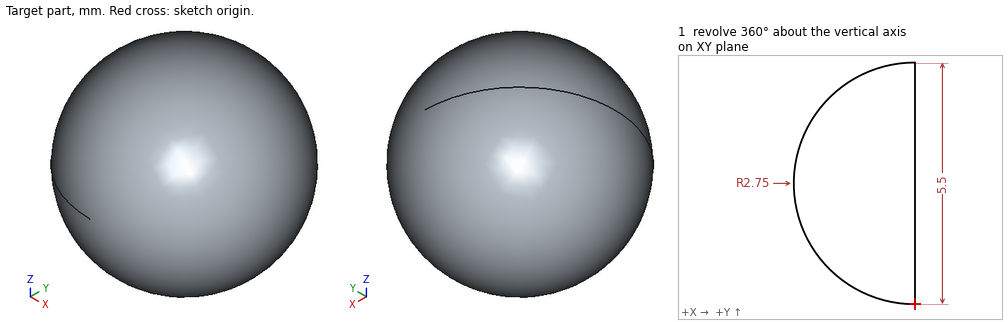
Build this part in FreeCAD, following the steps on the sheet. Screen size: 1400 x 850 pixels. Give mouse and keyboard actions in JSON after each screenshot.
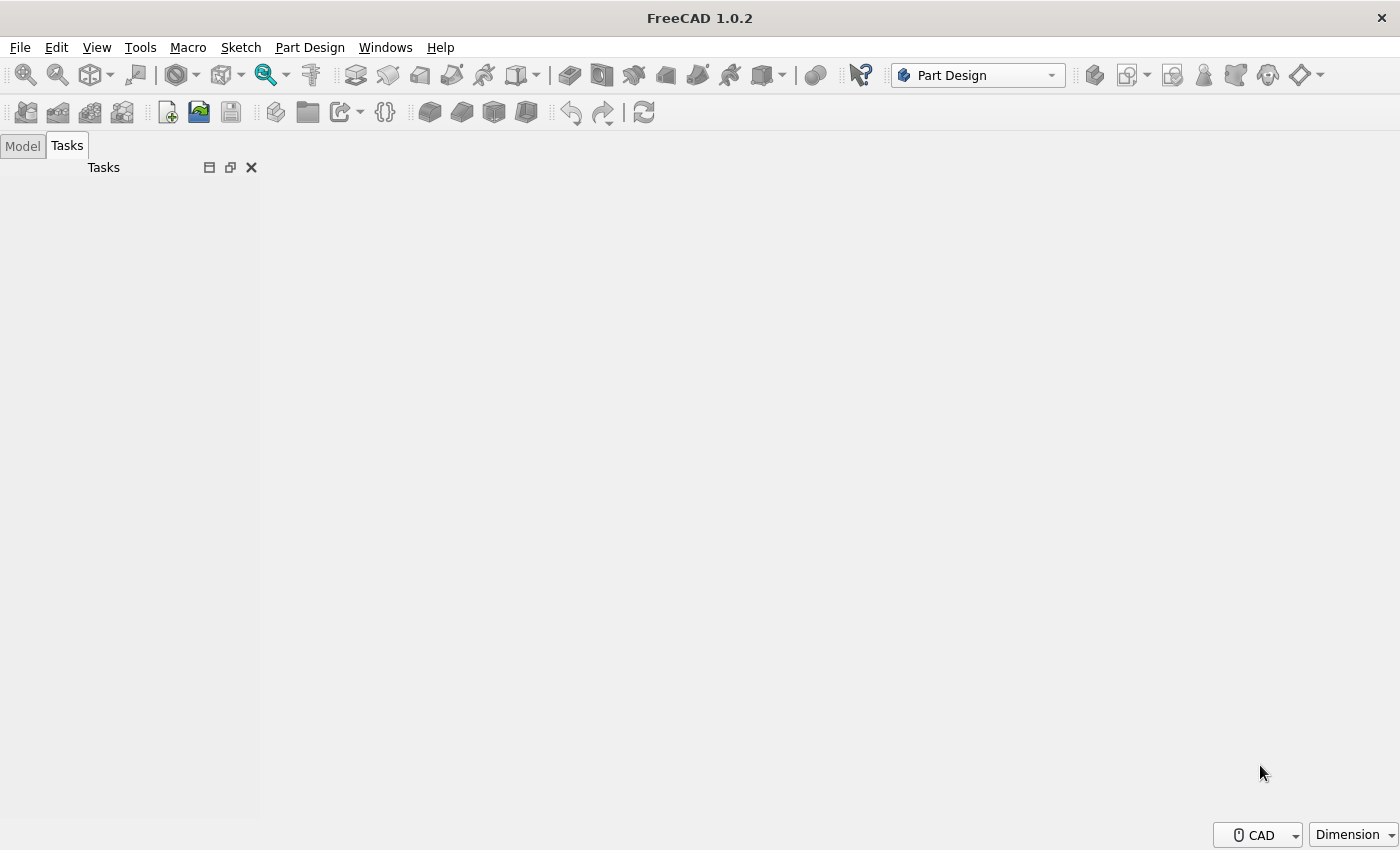
{"action": "left_click", "coordinate": [168, 112]}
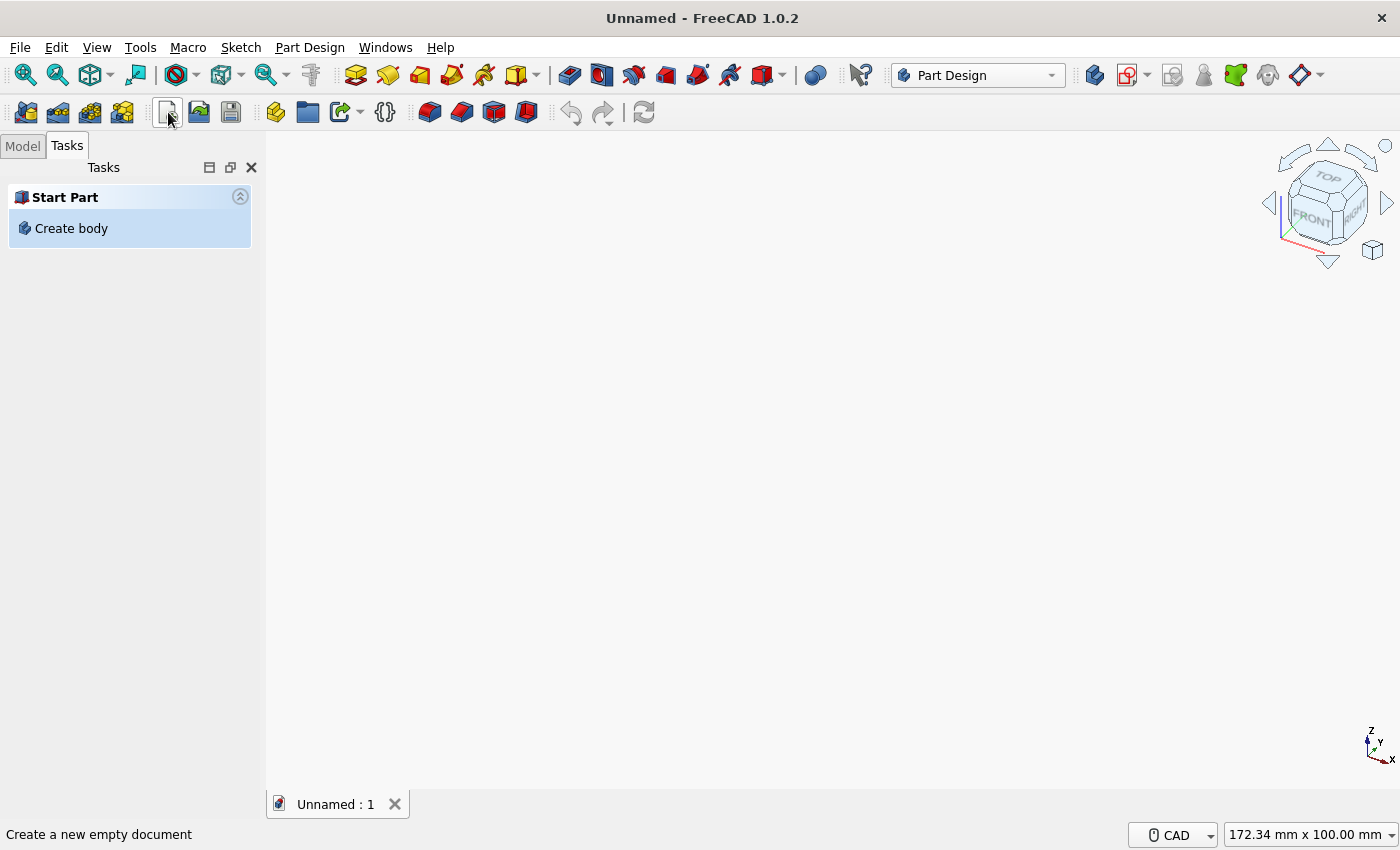
{"action": "left_click", "coordinate": [1128, 76]}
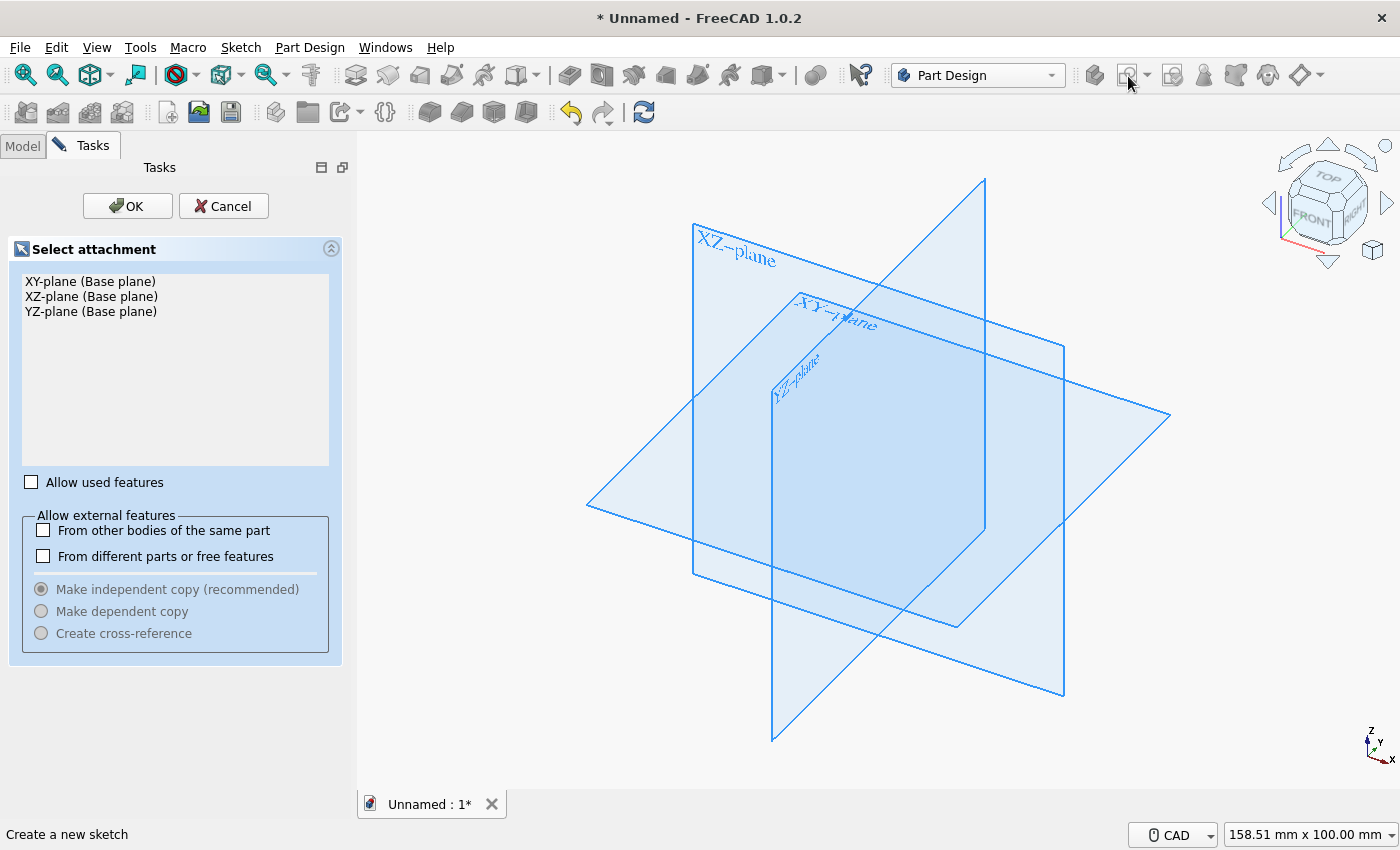
{"action": "left_click", "coordinate": [82, 282]}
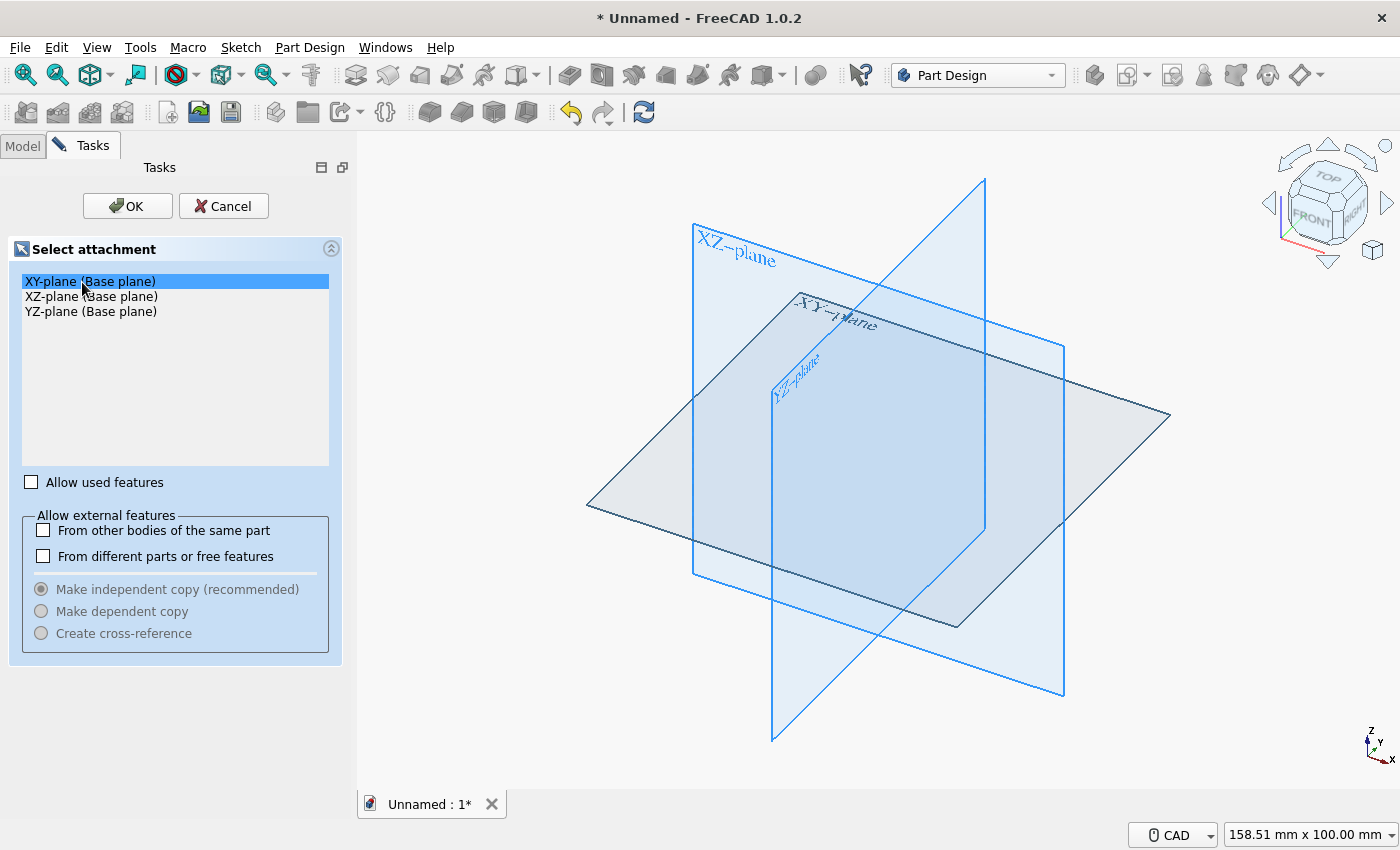
{"action": "left_click", "coordinate": [128, 206]}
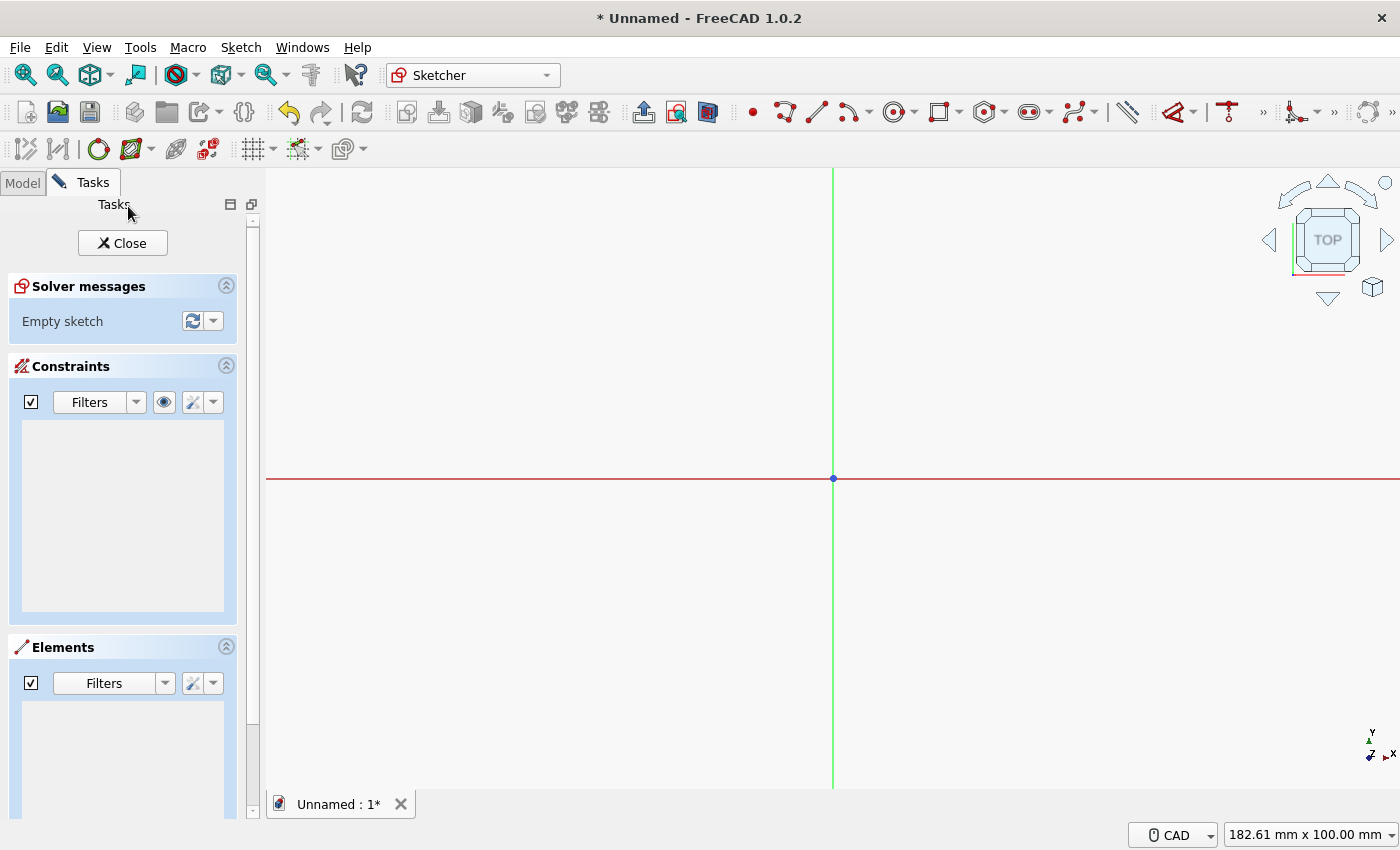
{"action": "scroll", "coordinate": [830, 460], "scroll_direction": "up", "scroll_amount": 12}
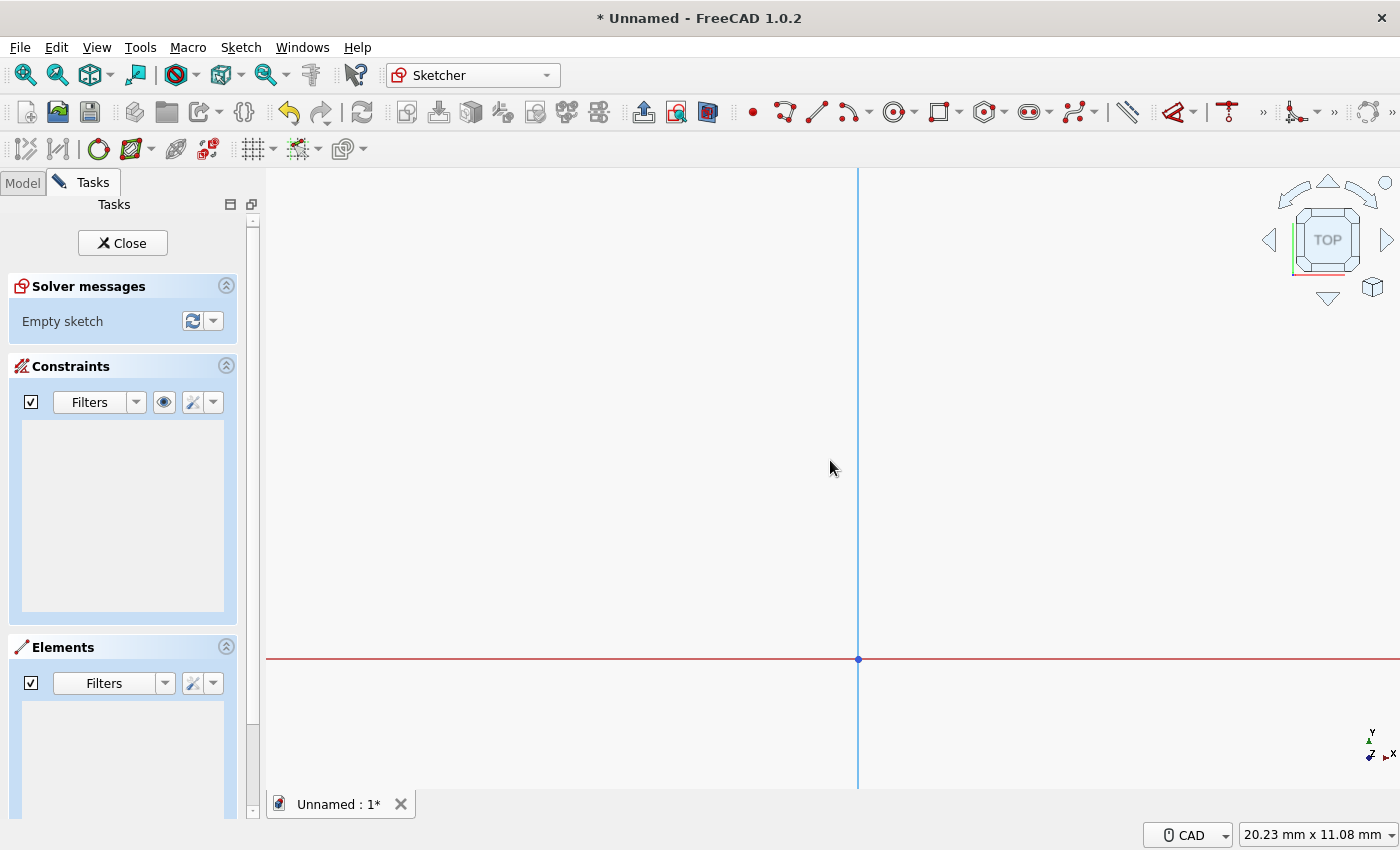
{"action": "left_click", "coordinate": [818, 112]}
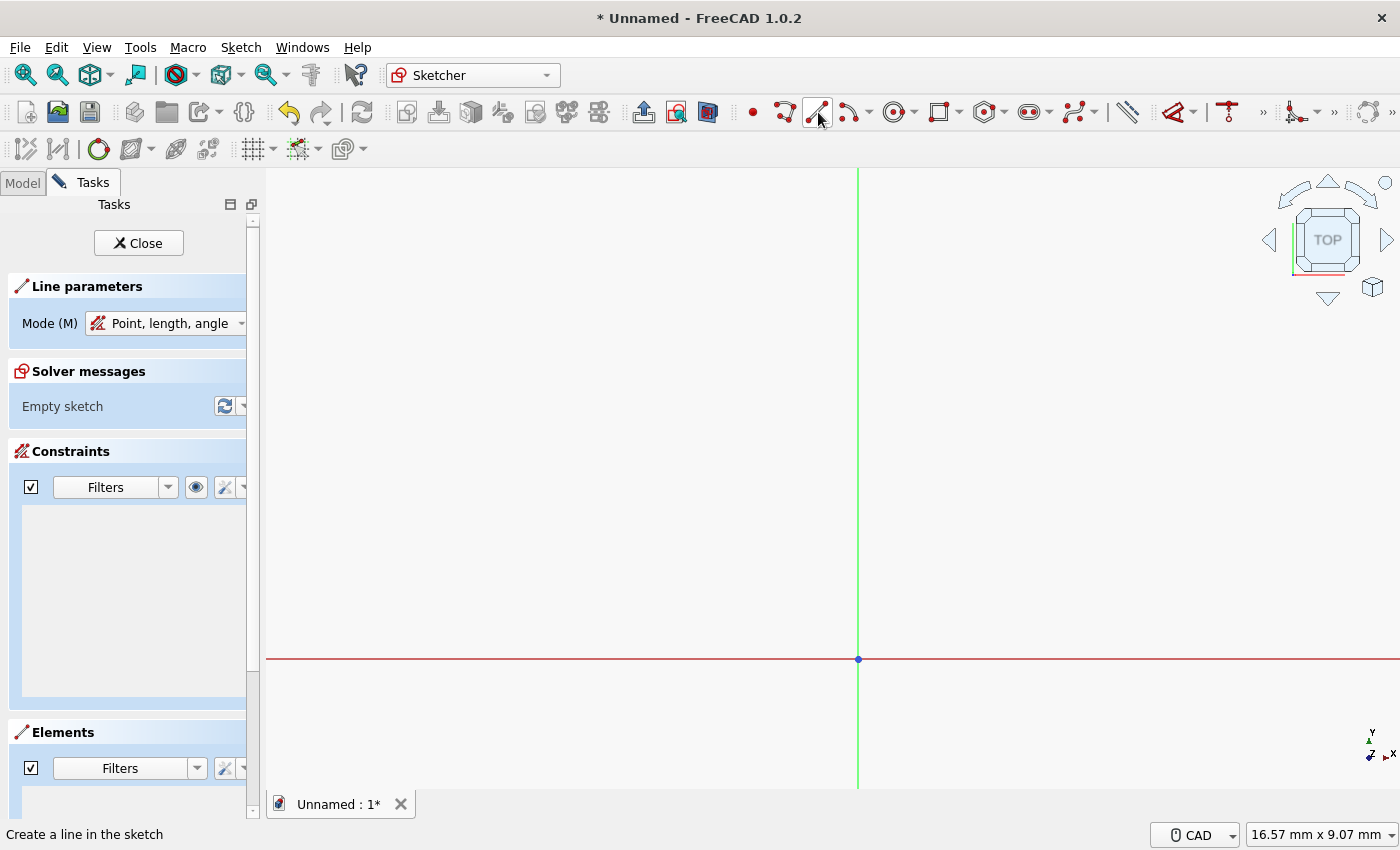
{"action": "left_click", "coordinate": [858, 659]}
{"action": "left_click", "coordinate": [849, 283]}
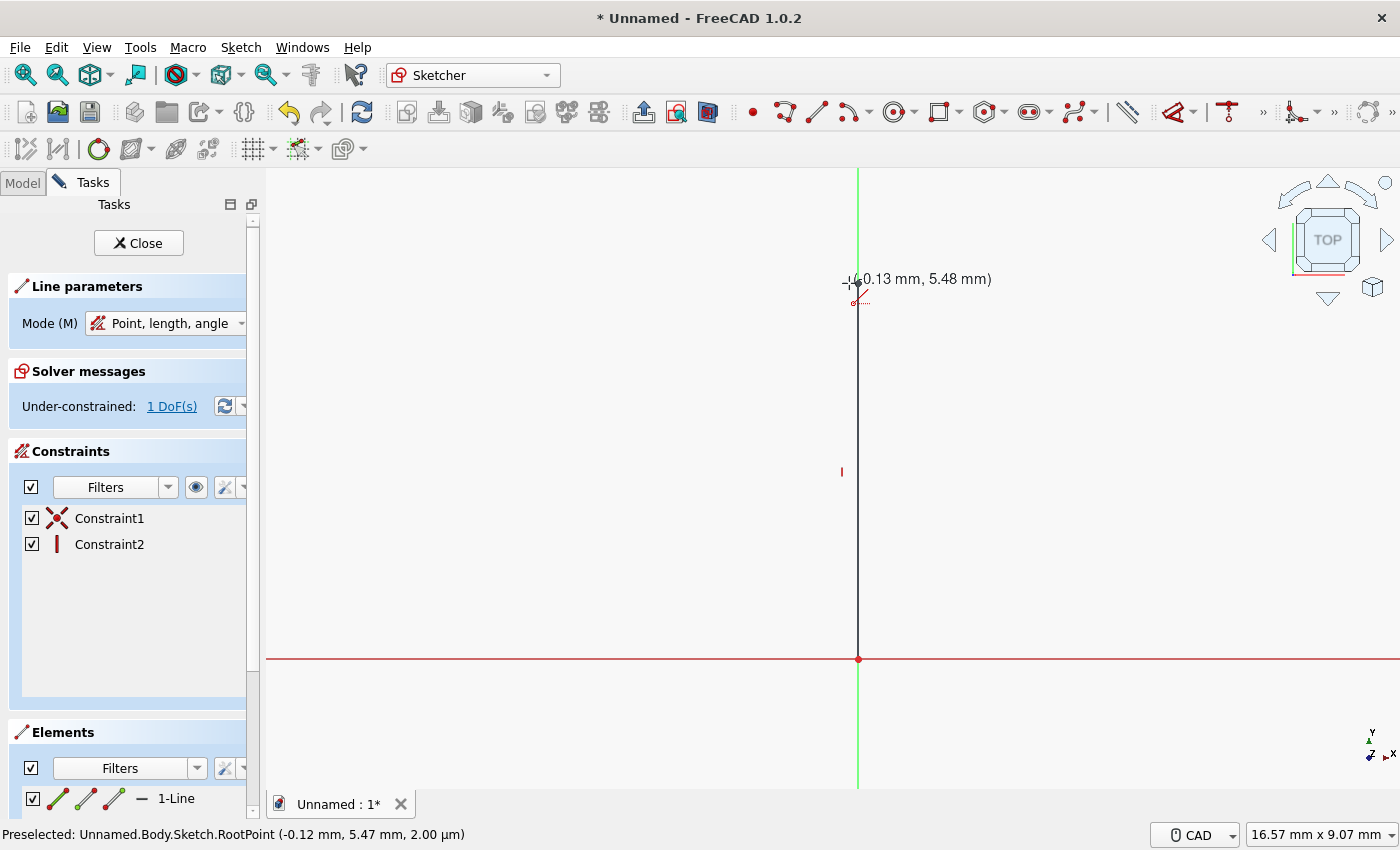
{"action": "key", "text": "g 3 a"}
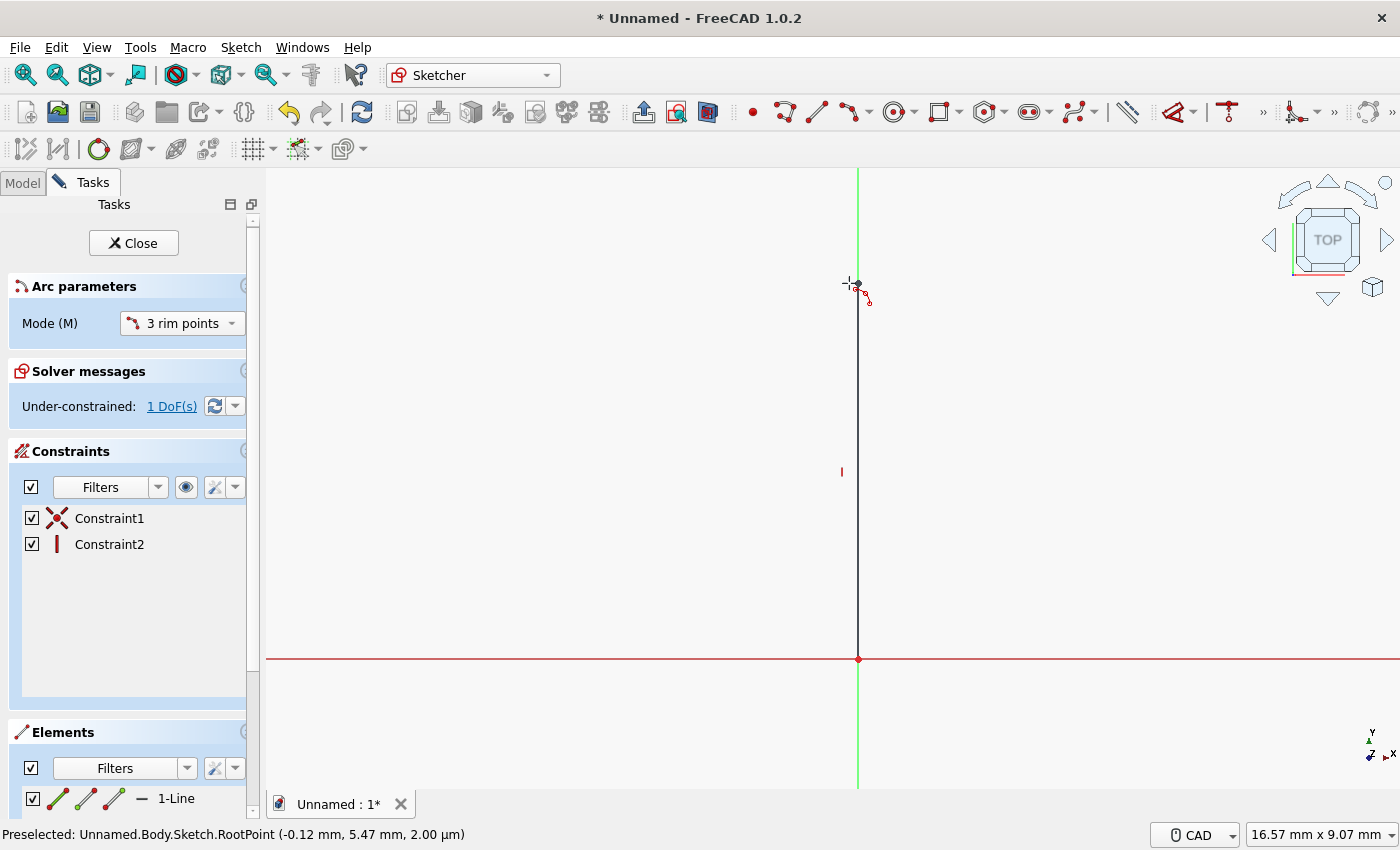
{"action": "left_click", "coordinate": [849, 283]}
{"action": "left_click", "coordinate": [858, 659]}
{"action": "left_click", "coordinate": [670, 471]}
{"action": "key", "text": "Escape"}